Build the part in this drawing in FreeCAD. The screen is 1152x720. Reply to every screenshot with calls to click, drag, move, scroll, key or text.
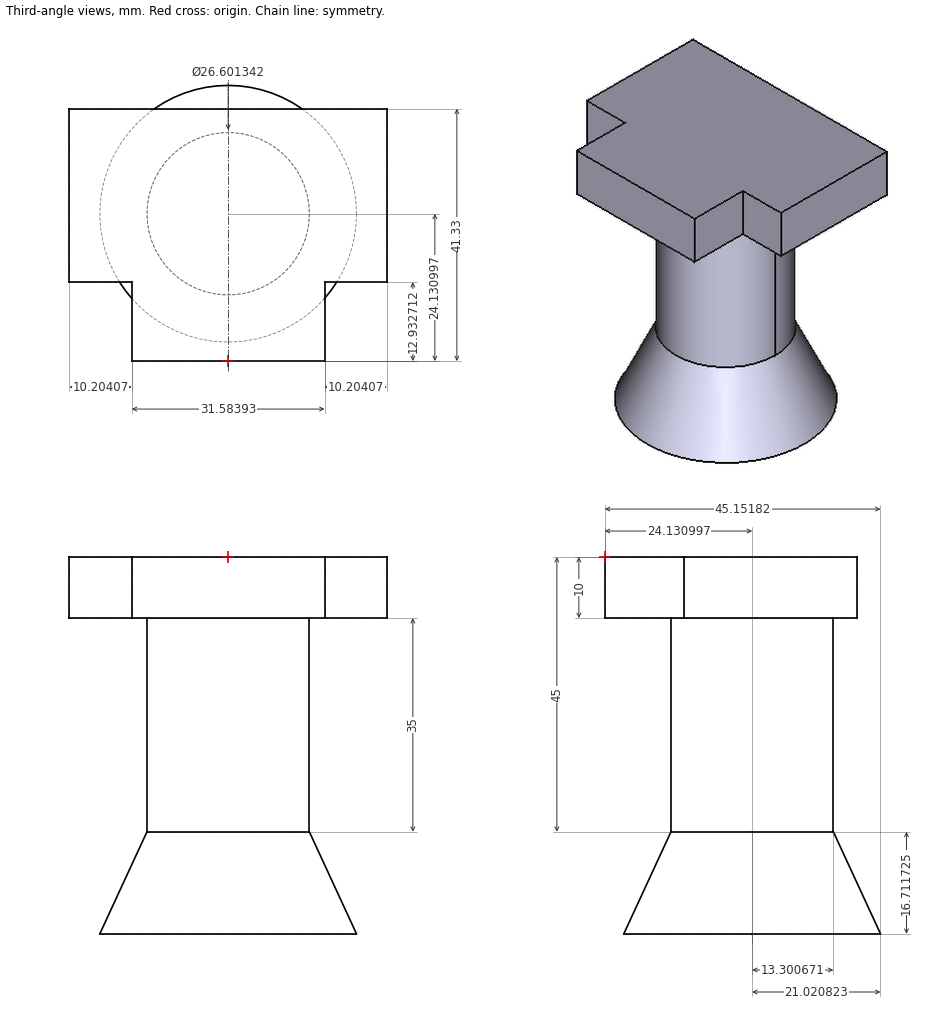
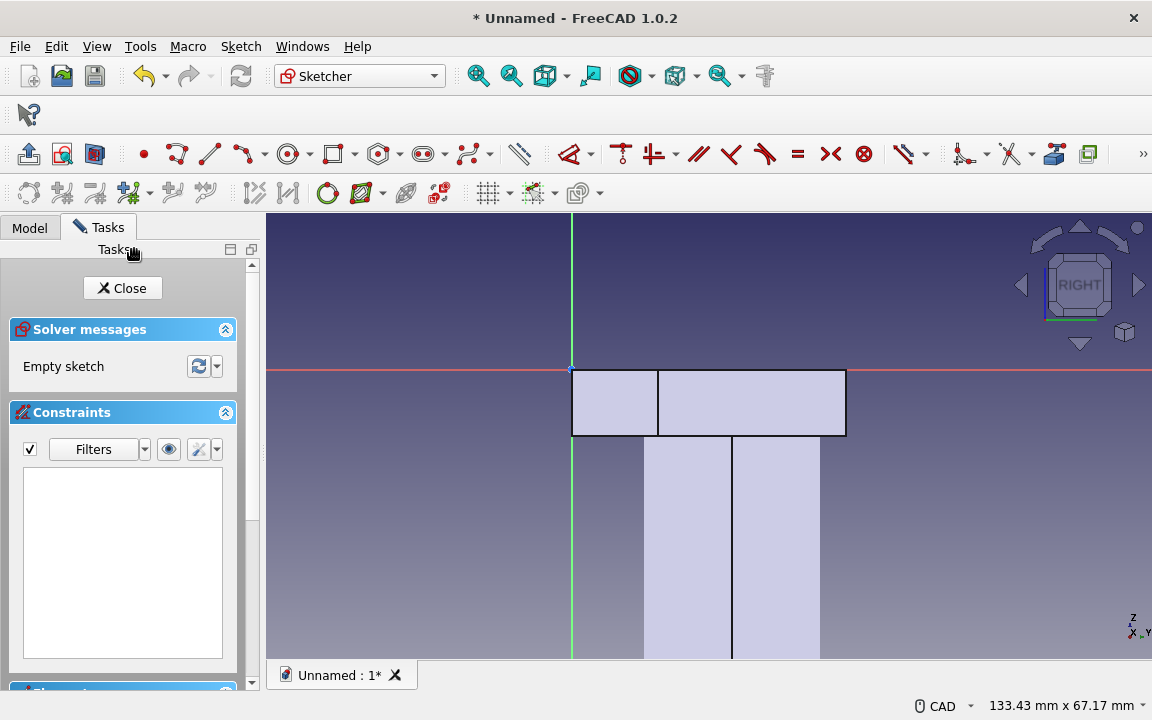
key(q)
key(s)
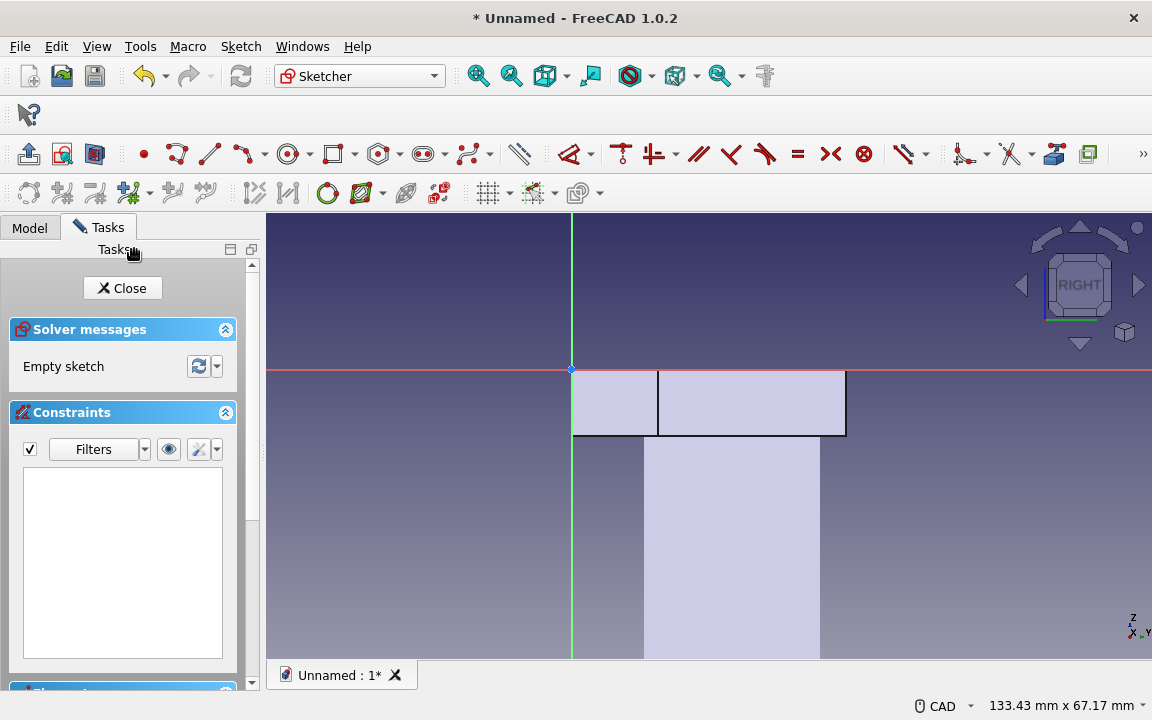
scroll(640, 436, down, 5)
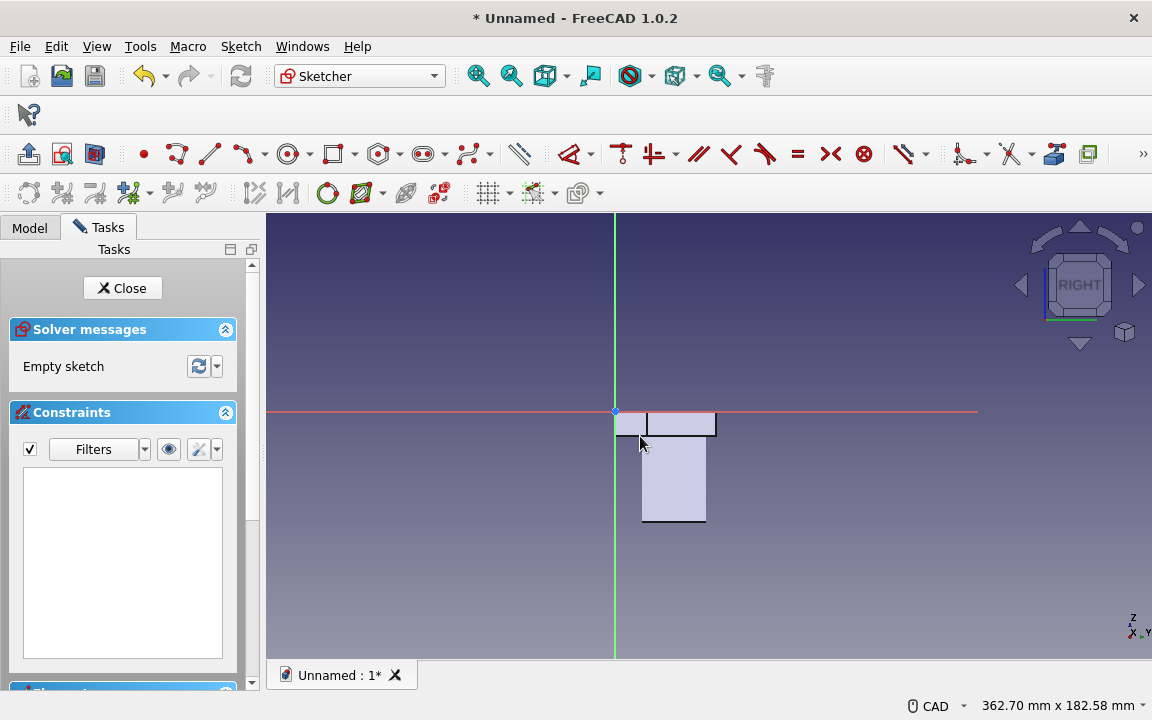
scroll(715, 579, up, 8)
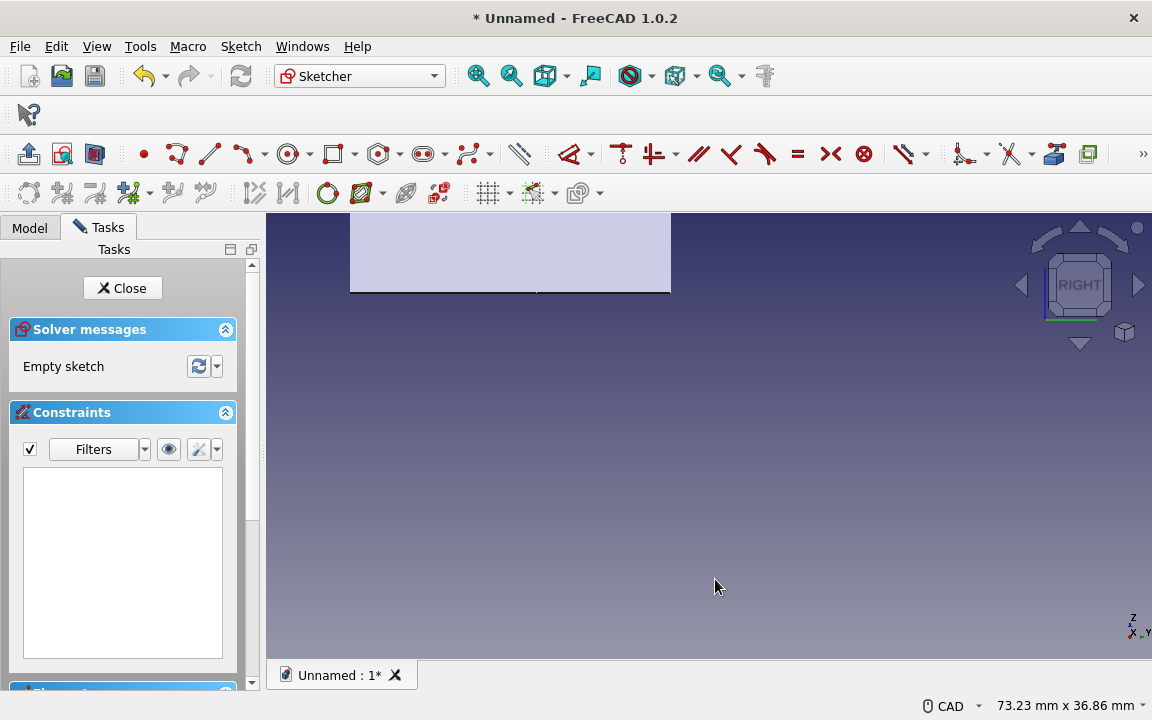
click(177, 154)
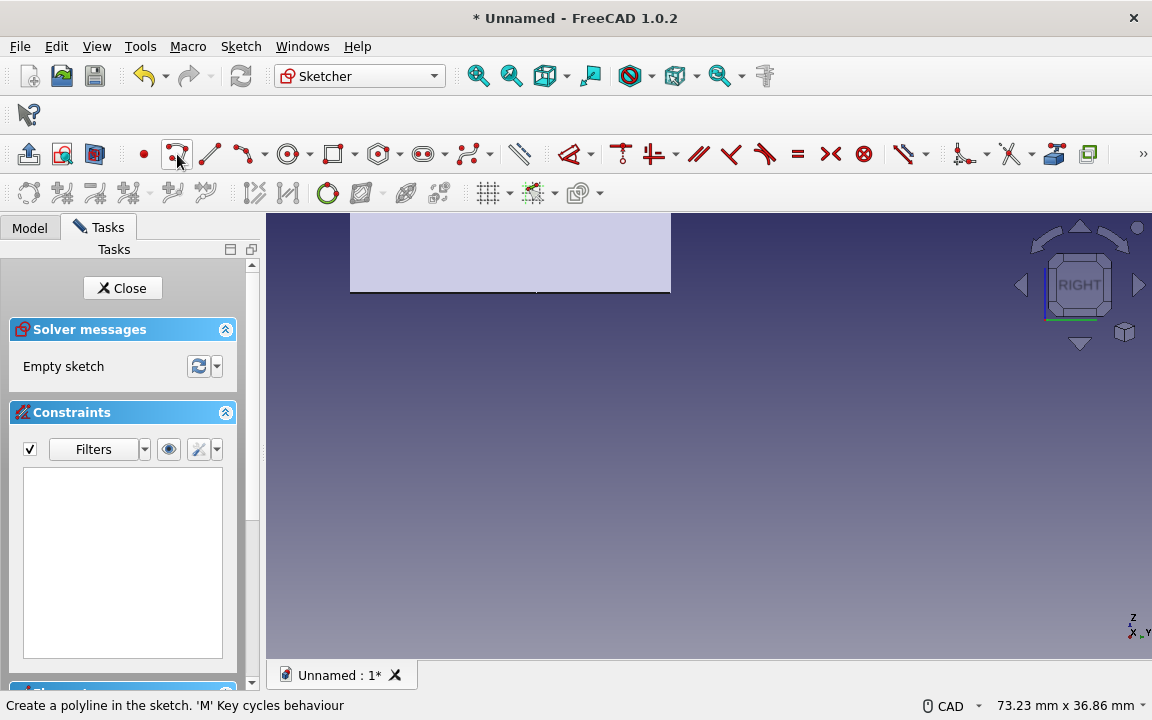
click(511, 293)
click(511, 495)
click(765, 495)
click(671, 293)
click(511, 294)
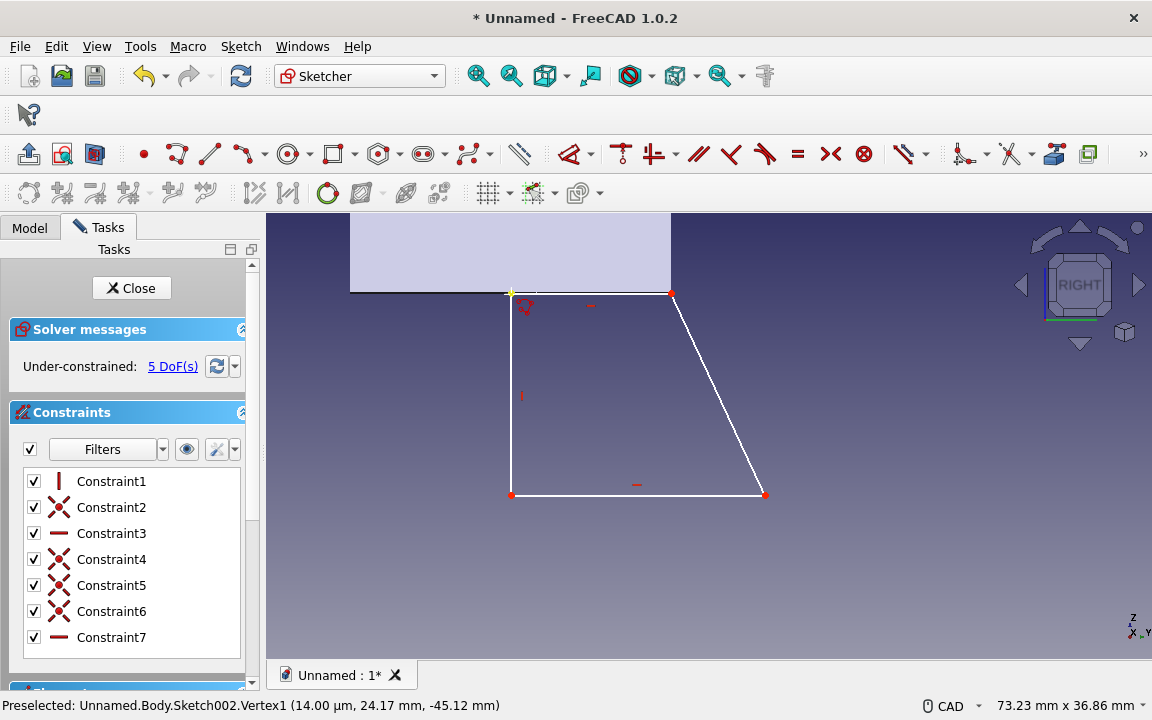
click(210, 154)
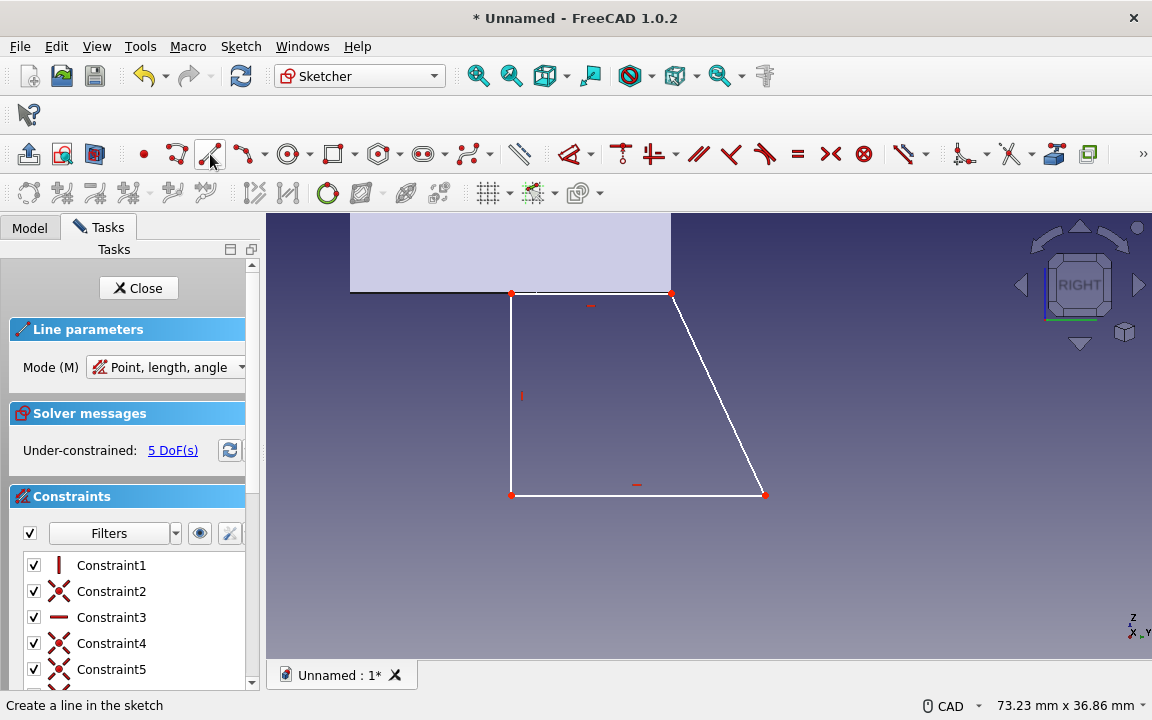
click(511, 515)
click(511, 576)
key(Escape)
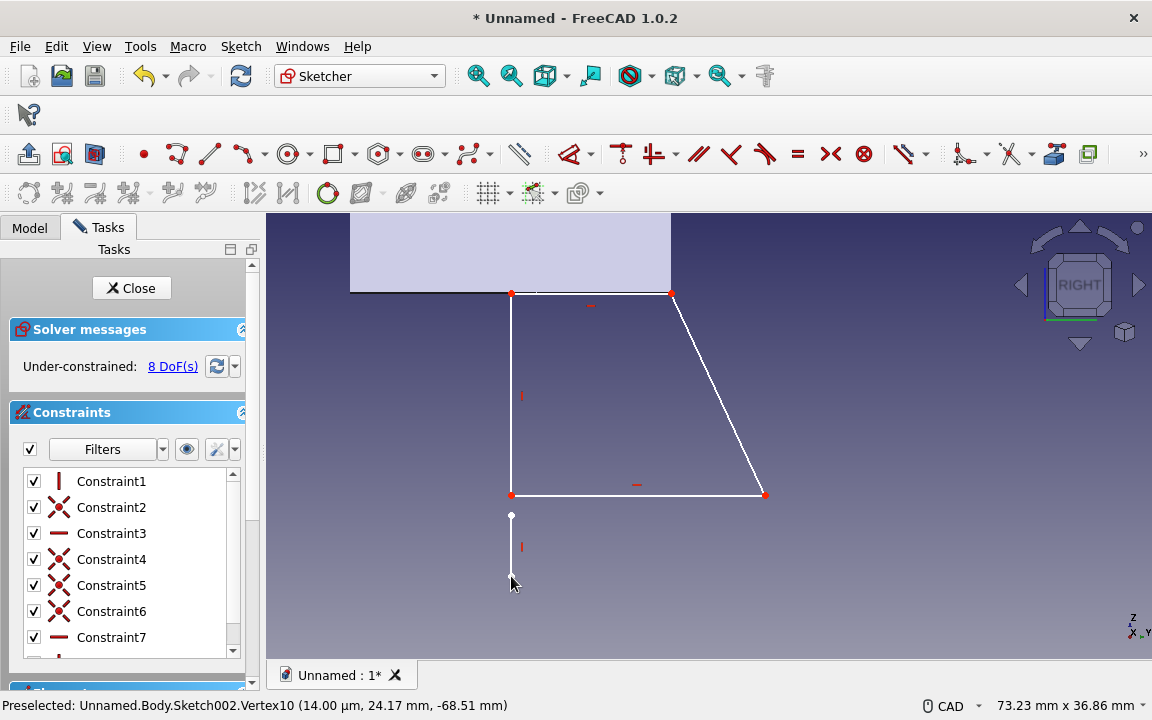
click(511, 534)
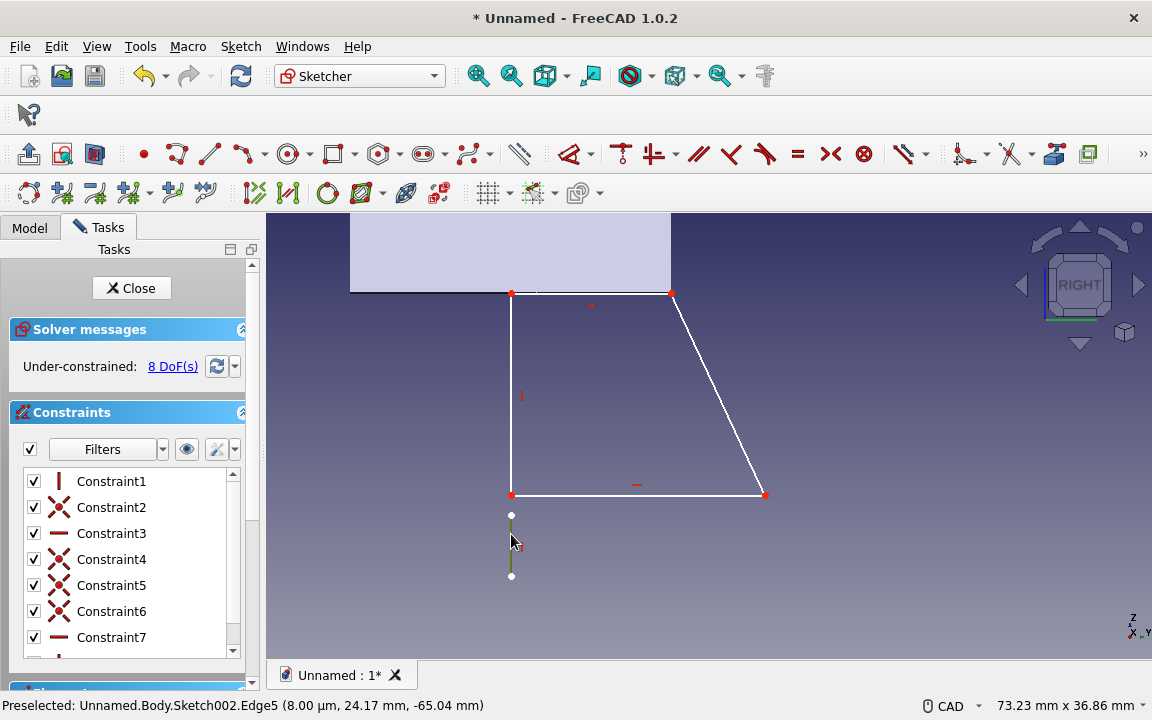
click(520, 154)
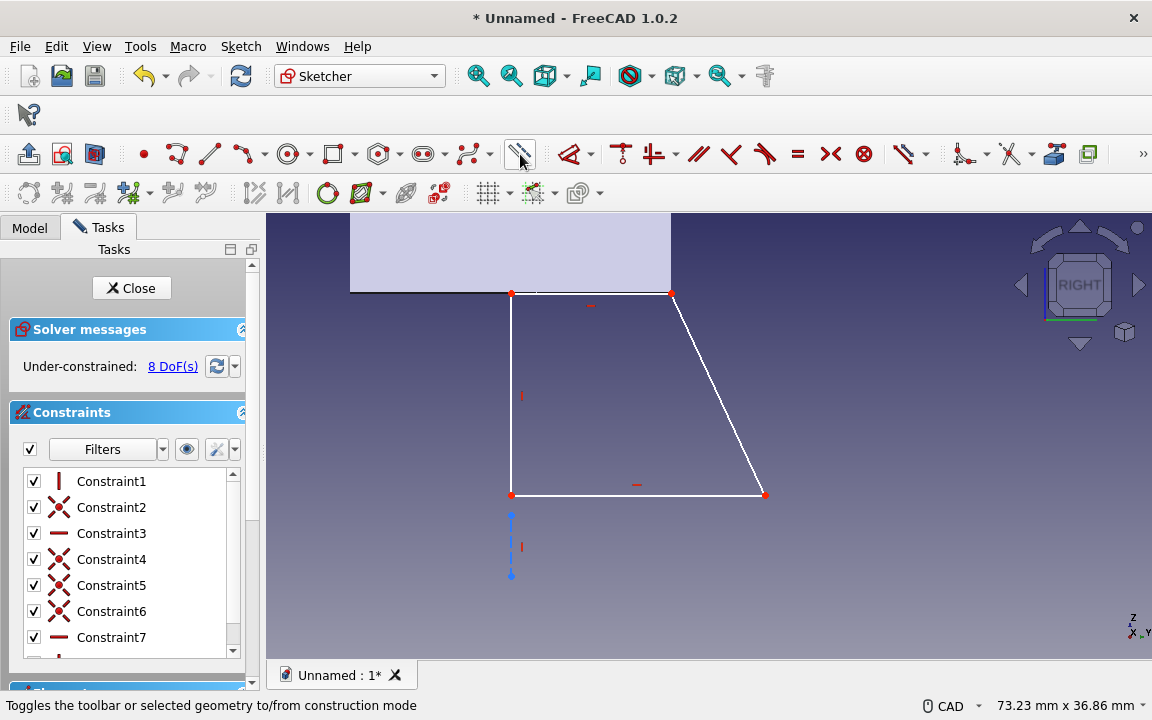
click(568, 154)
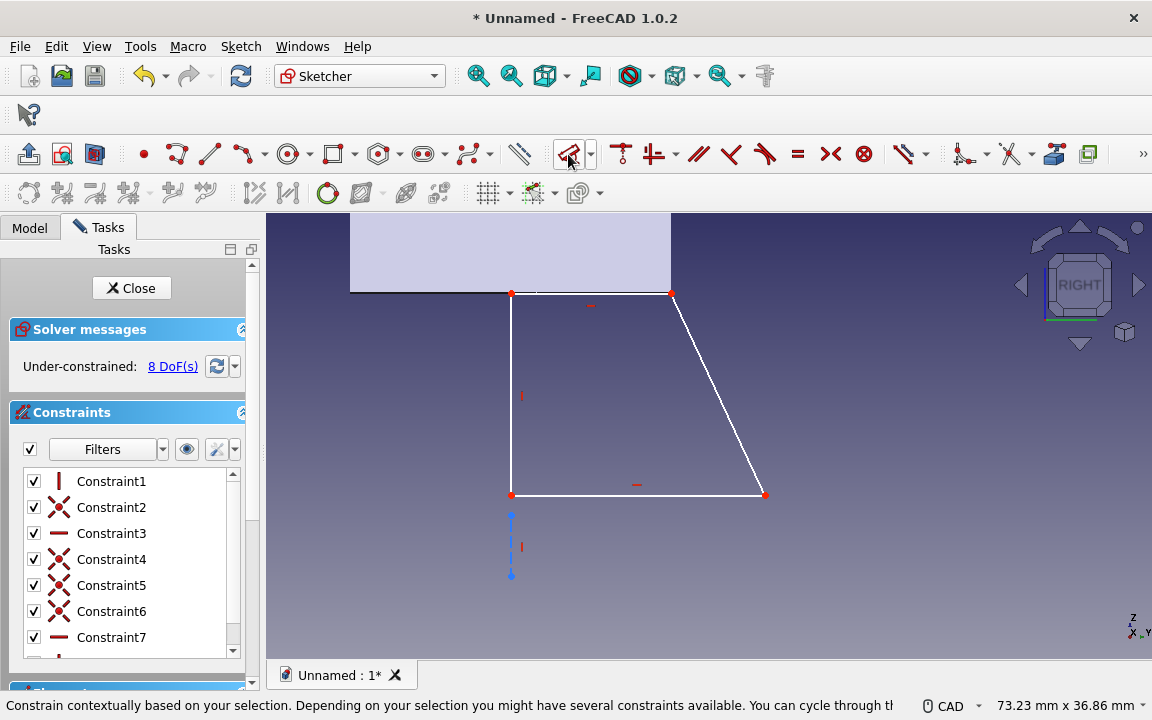
click(511, 294)
click(545, 268)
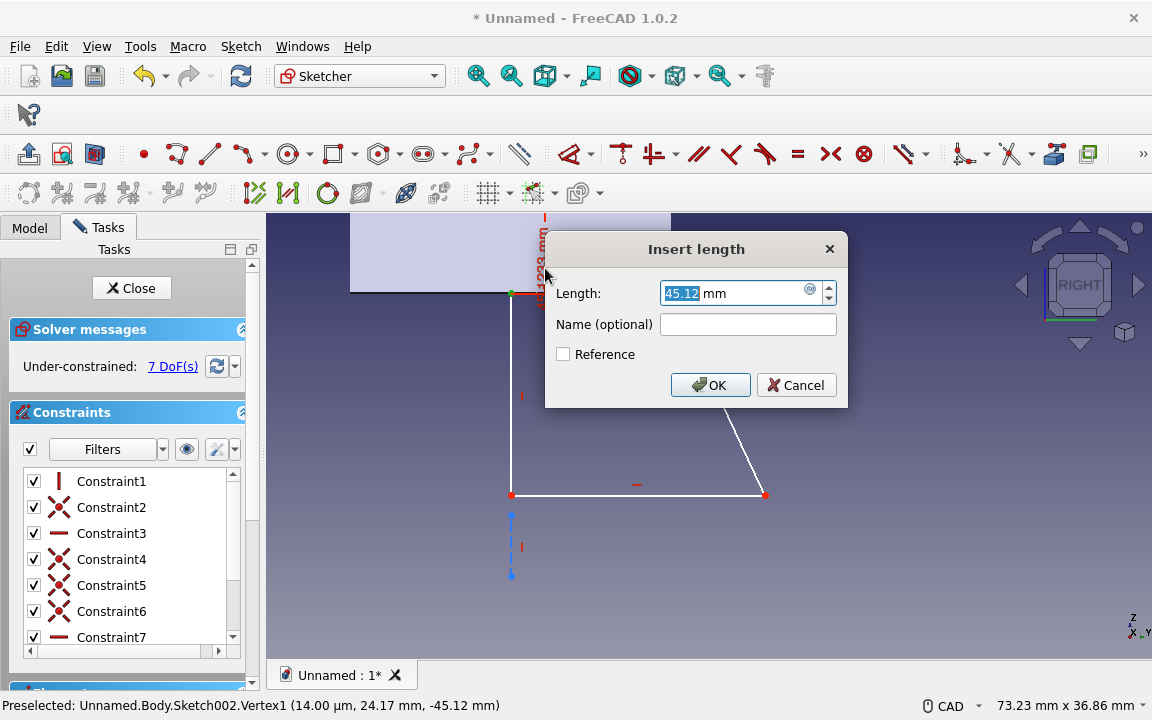
text(45)
key(Return)